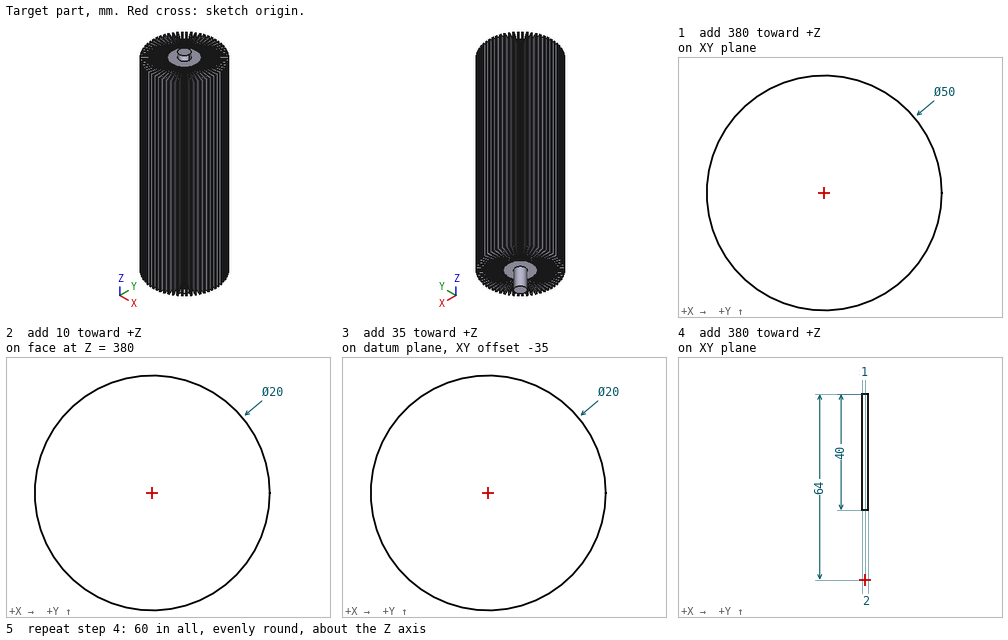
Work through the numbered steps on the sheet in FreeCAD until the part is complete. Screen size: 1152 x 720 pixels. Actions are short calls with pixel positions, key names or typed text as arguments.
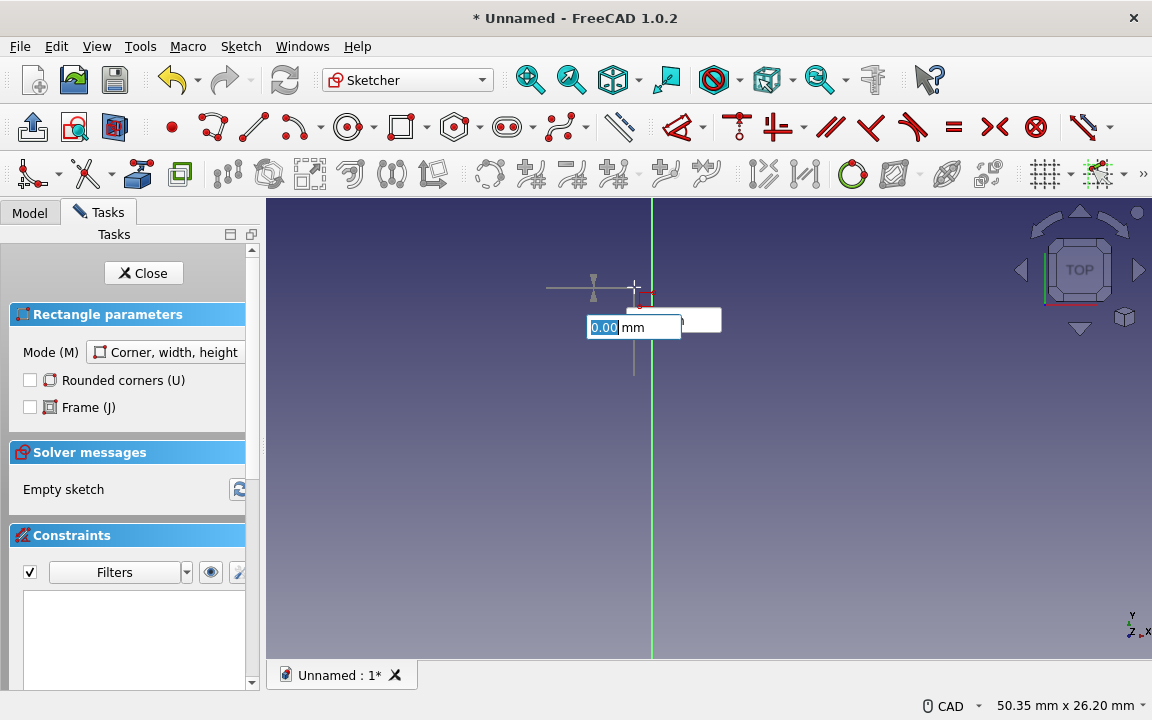
scroll(637, 291, down, 7)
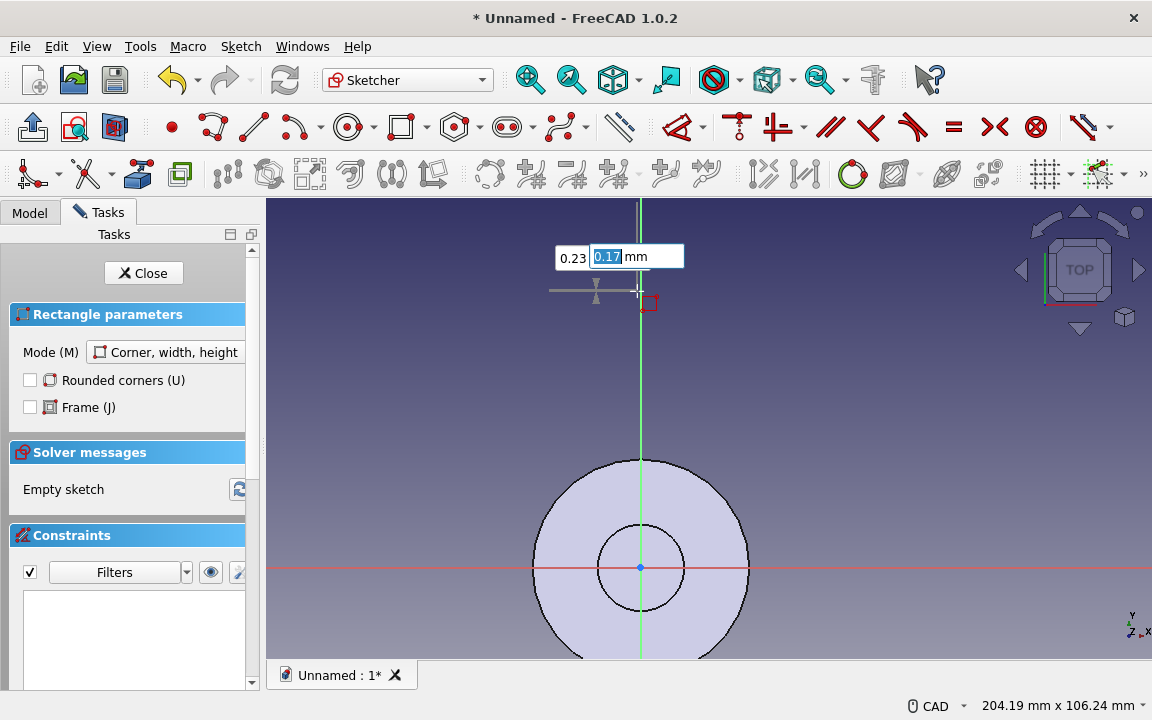
scroll(645, 464, up, 7)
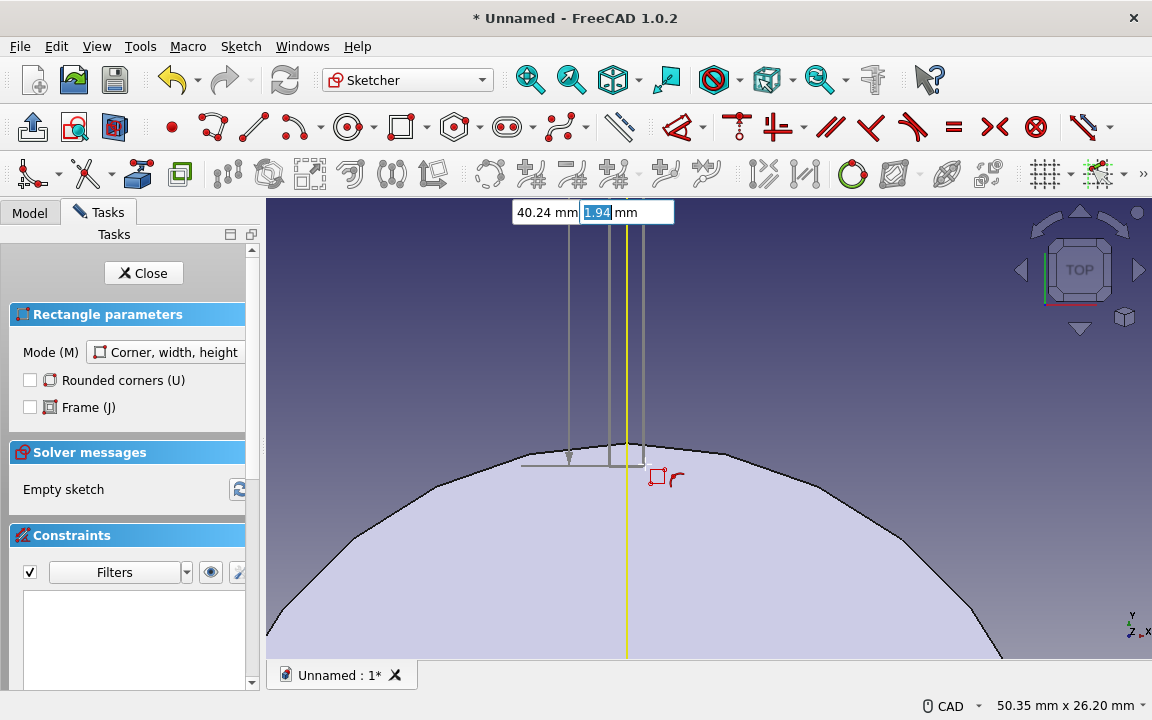
click(645, 461)
key(Escape)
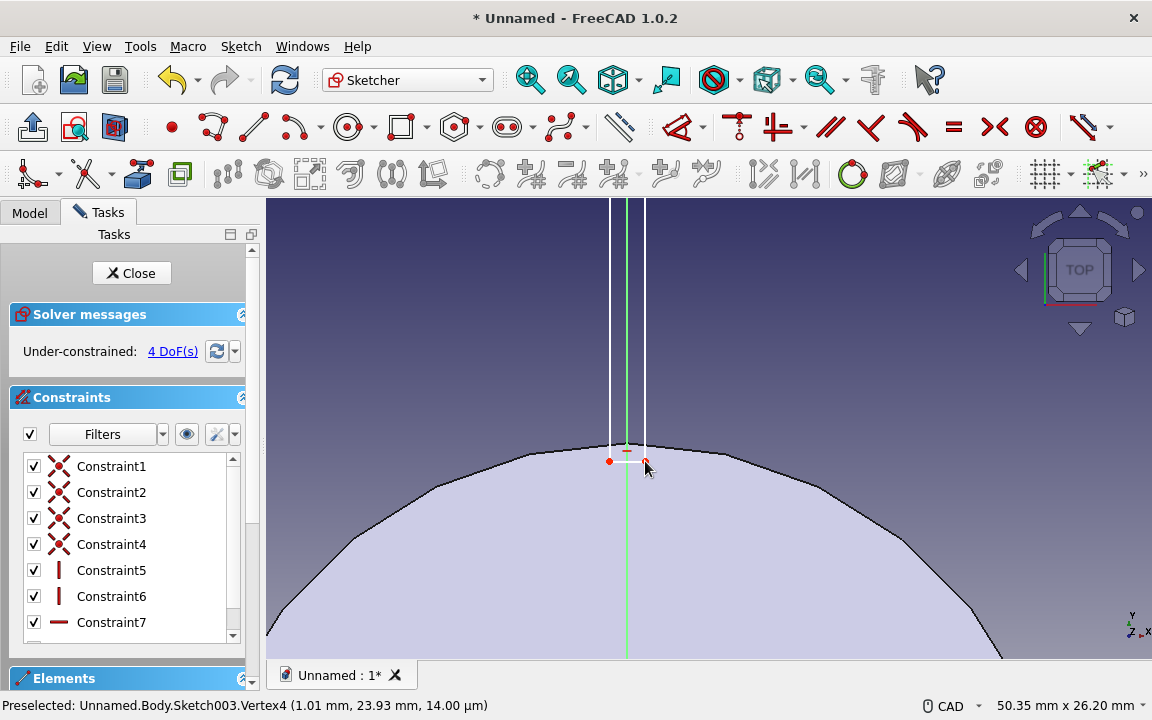
key(d)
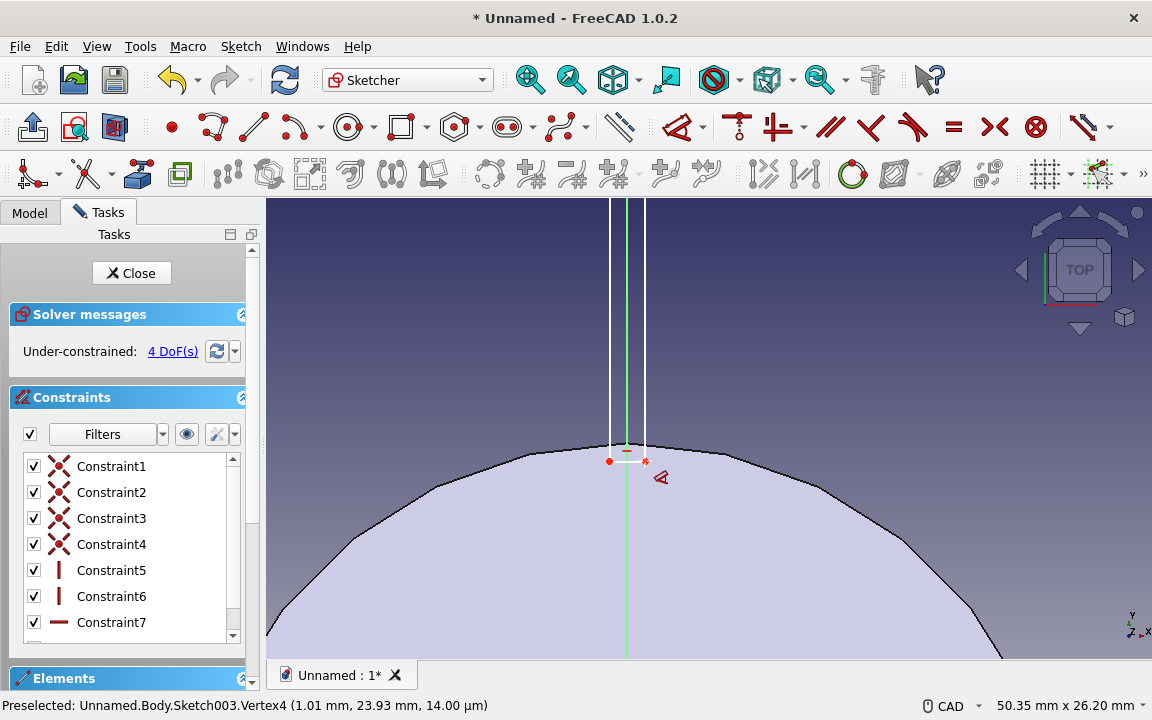
click(624, 462)
click(619, 496)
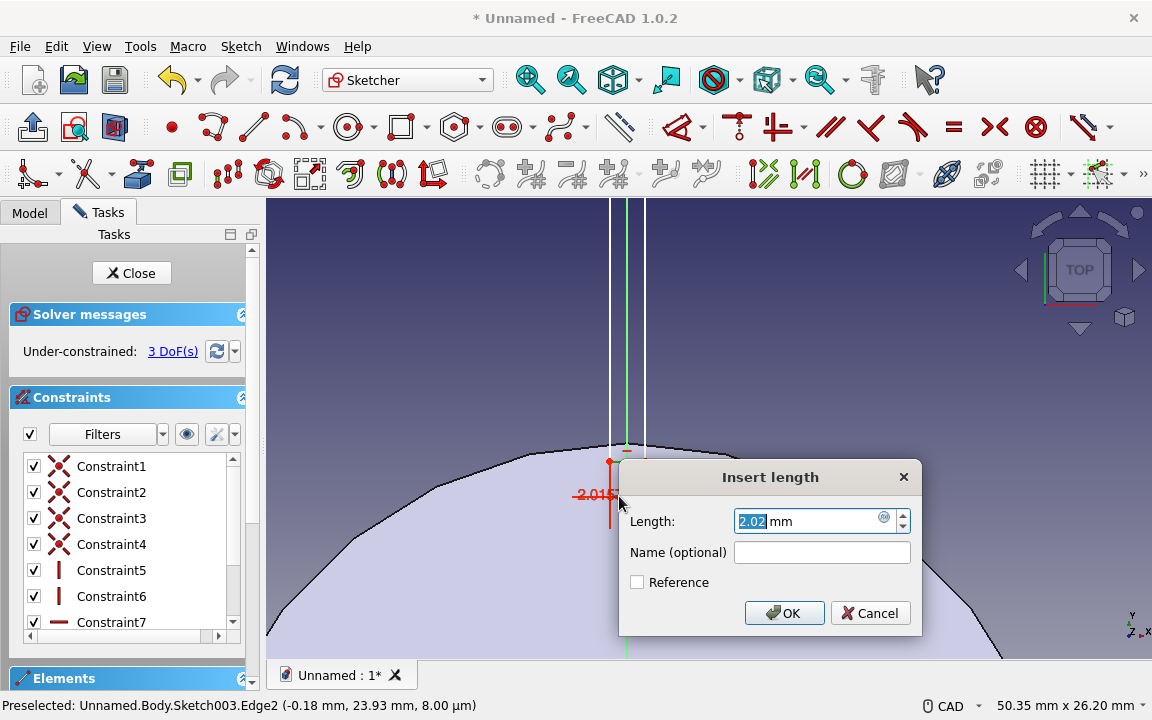
text(2)
key(Return)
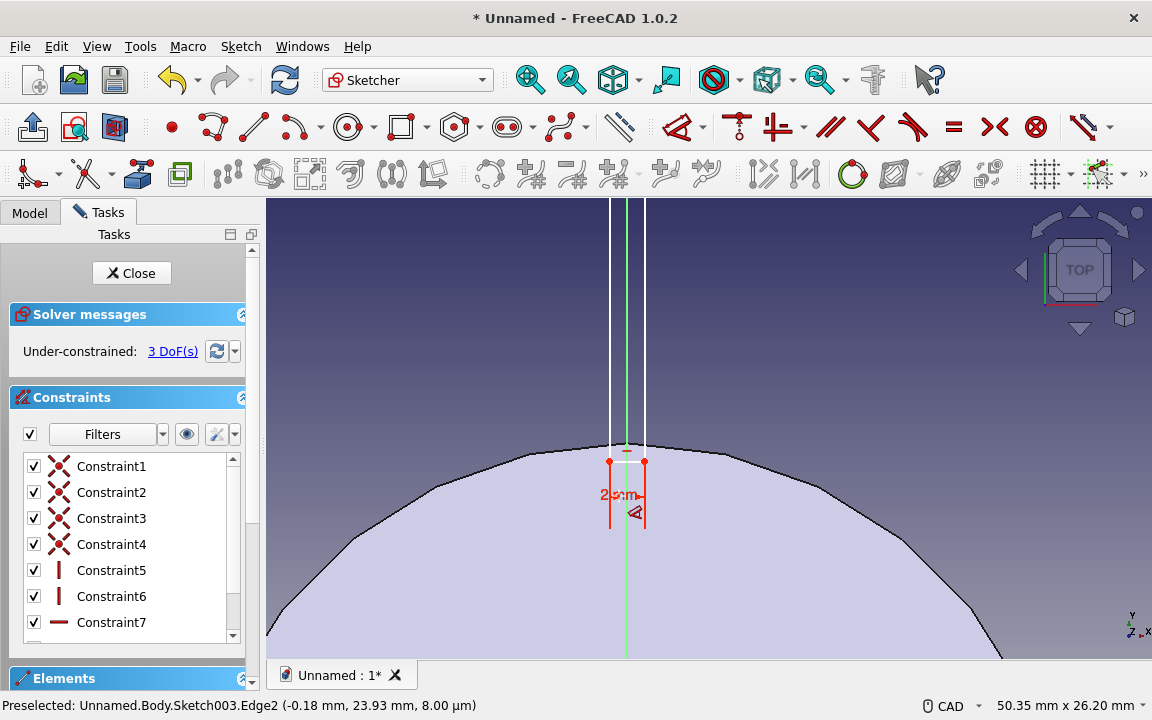
click(610, 251)
click(576, 344)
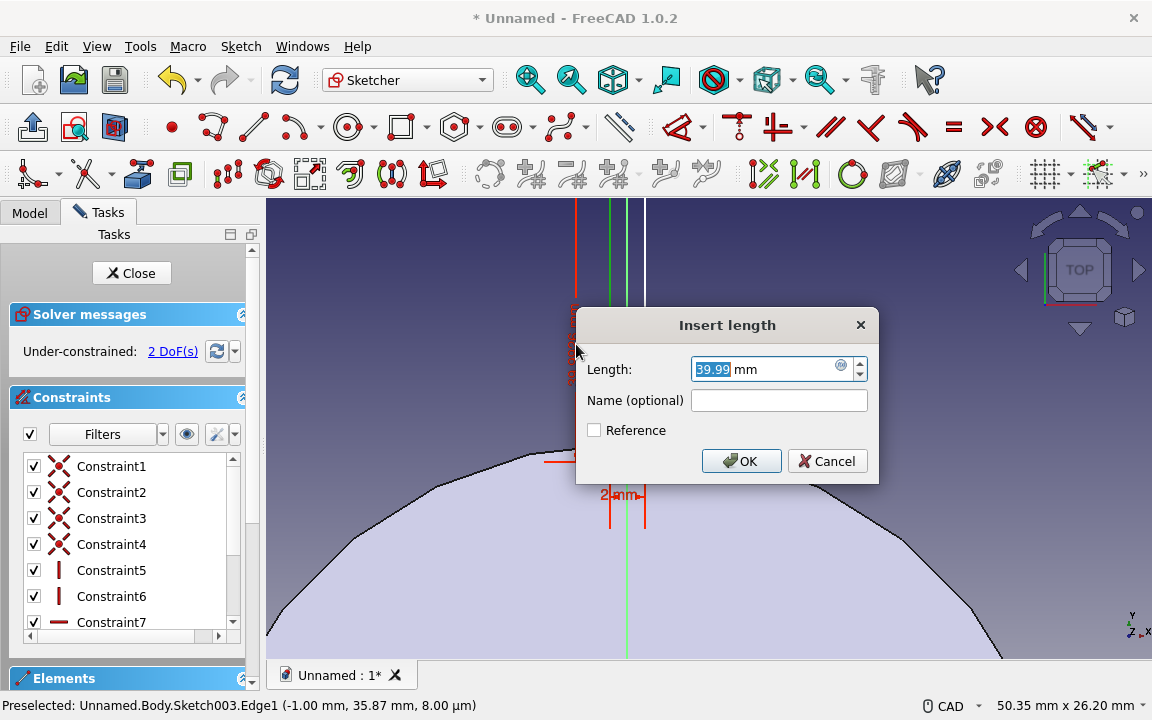
text(40)
key(Return)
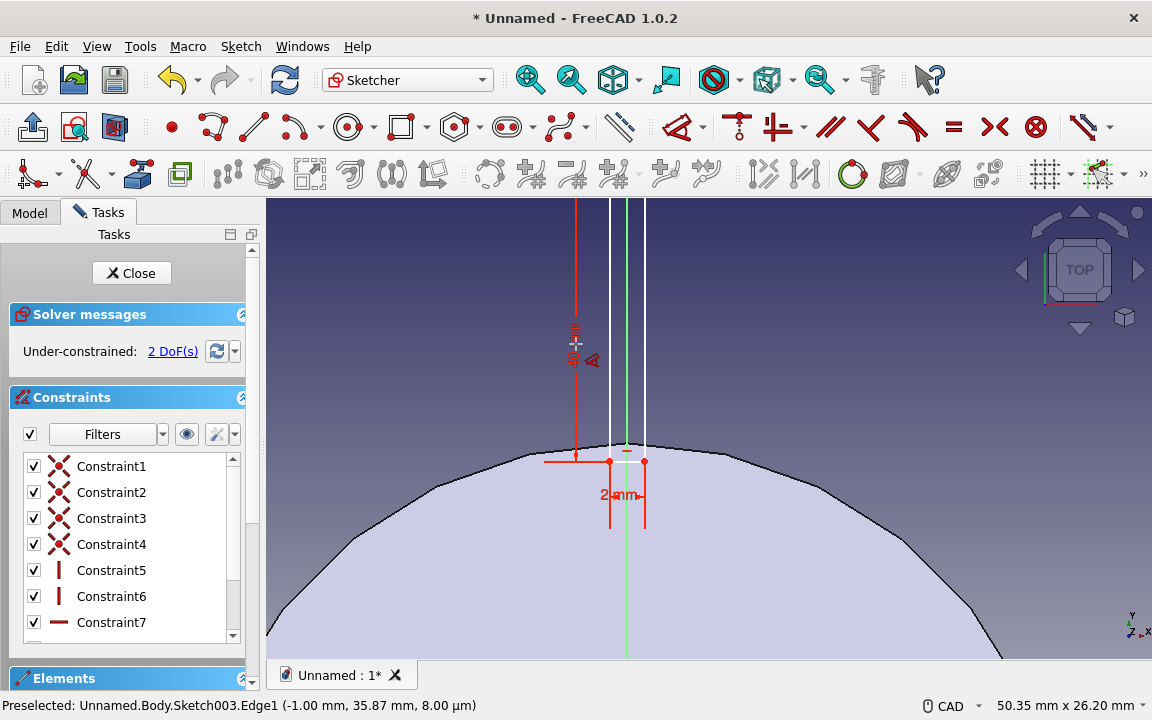
scroll(645, 464, down, 7)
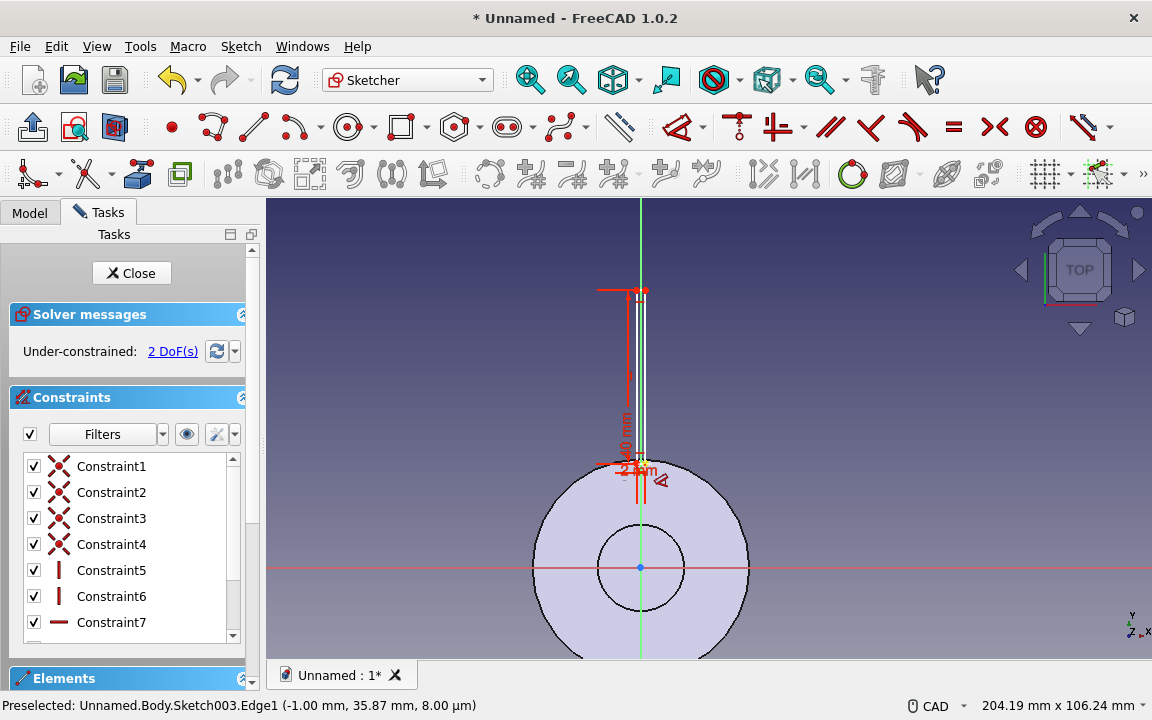
scroll(637, 290, up, 12)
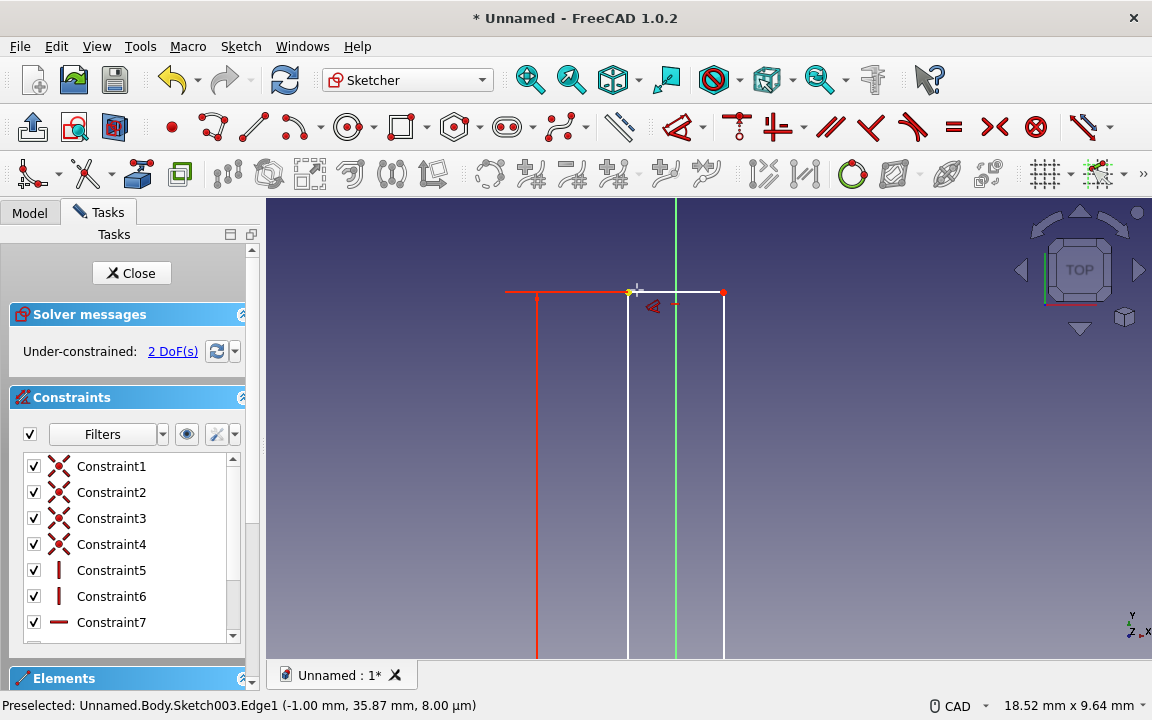
click(628, 292)
click(652, 258)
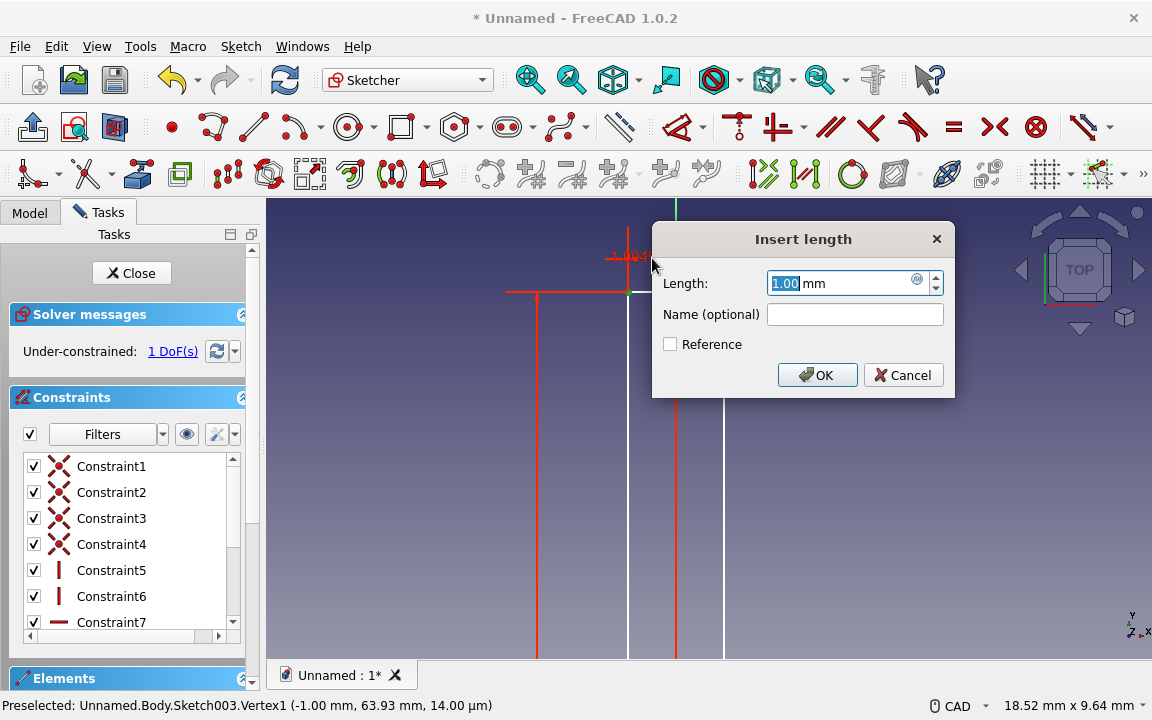
text(1)
key(Return)